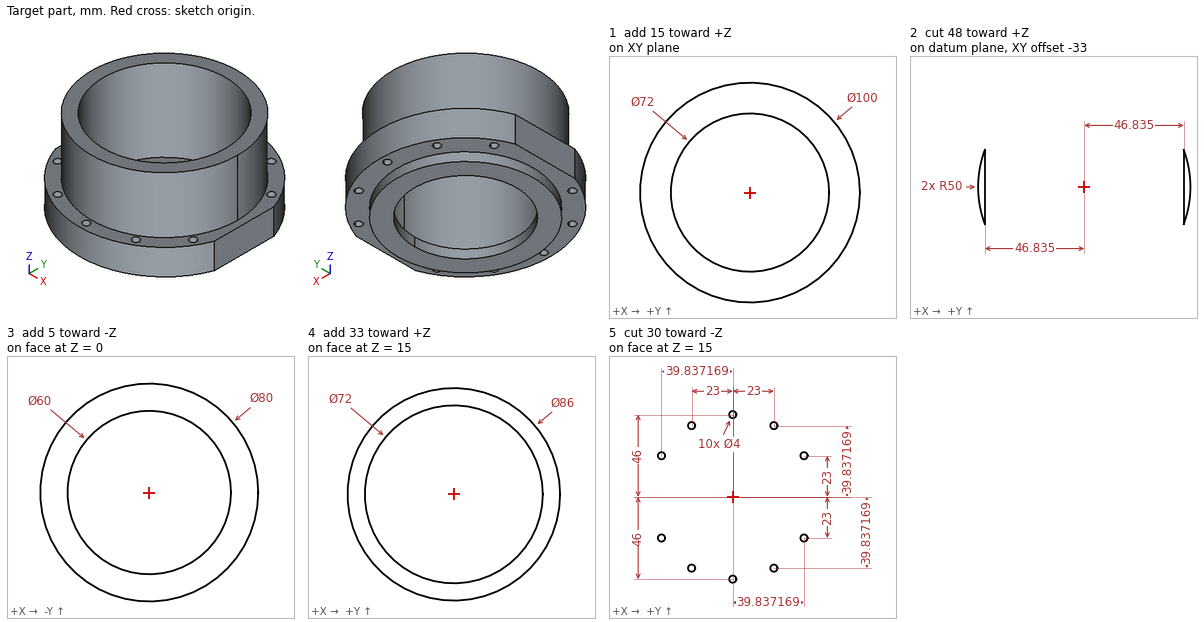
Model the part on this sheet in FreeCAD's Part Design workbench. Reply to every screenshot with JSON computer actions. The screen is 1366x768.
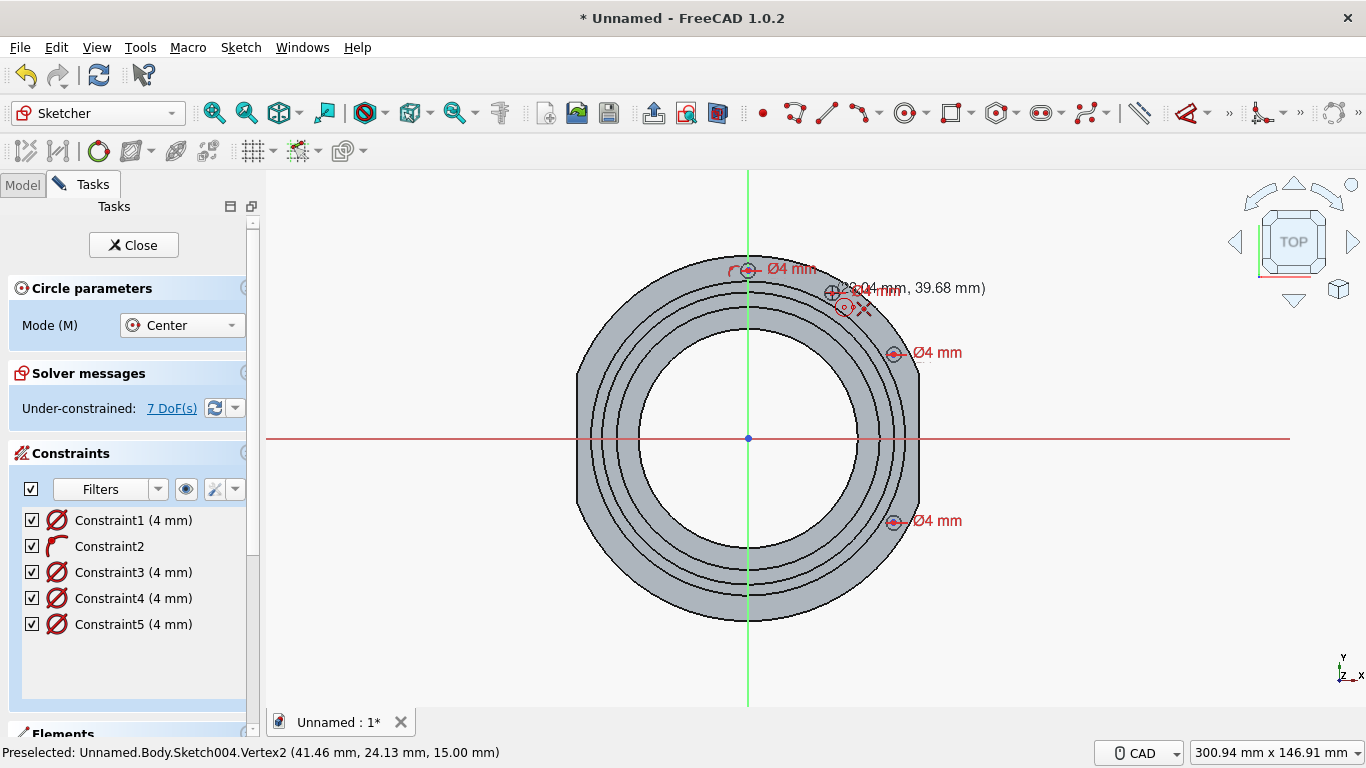
{"action": "scroll", "coordinate": [664, 293], "scroll_direction": "up", "scroll_amount": 6}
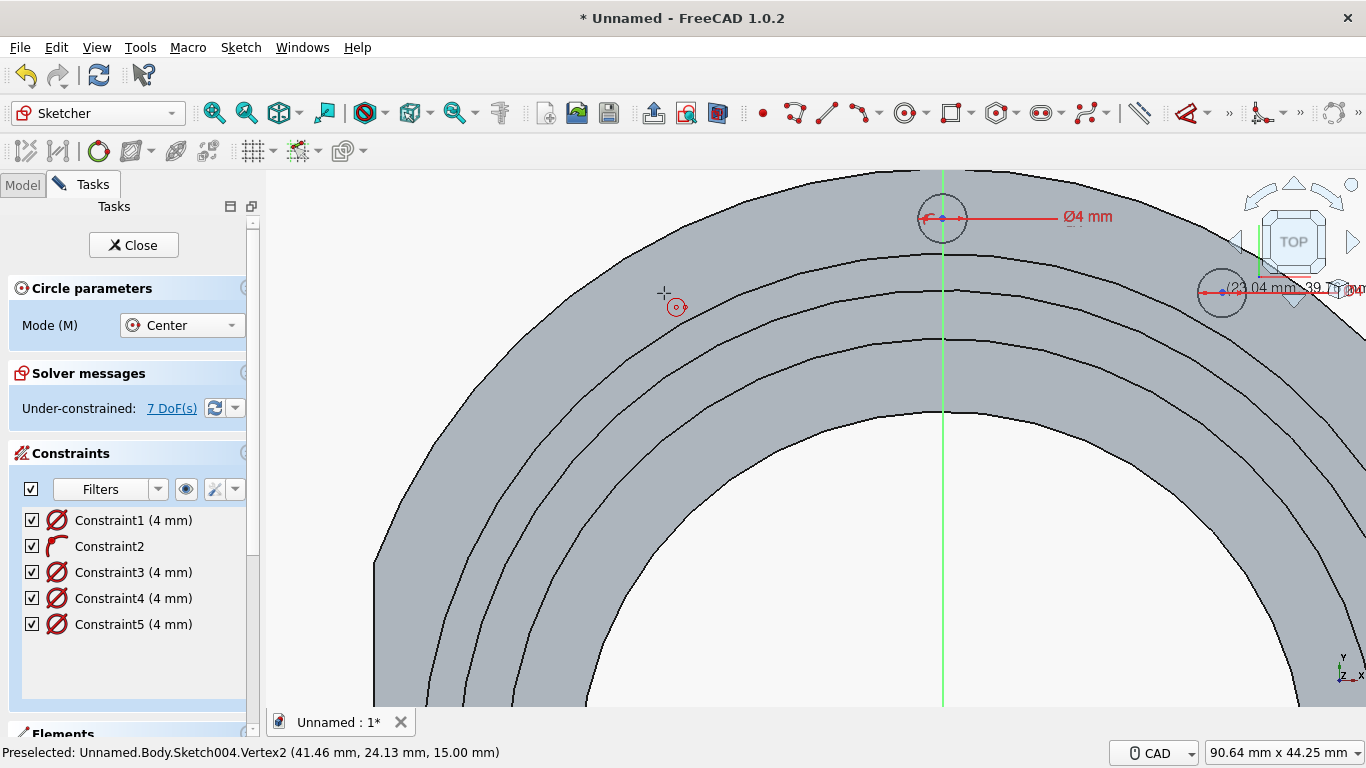
{"action": "left_click", "coordinate": [663, 292]}
{"action": "mouse_move", "coordinate": [681, 275]}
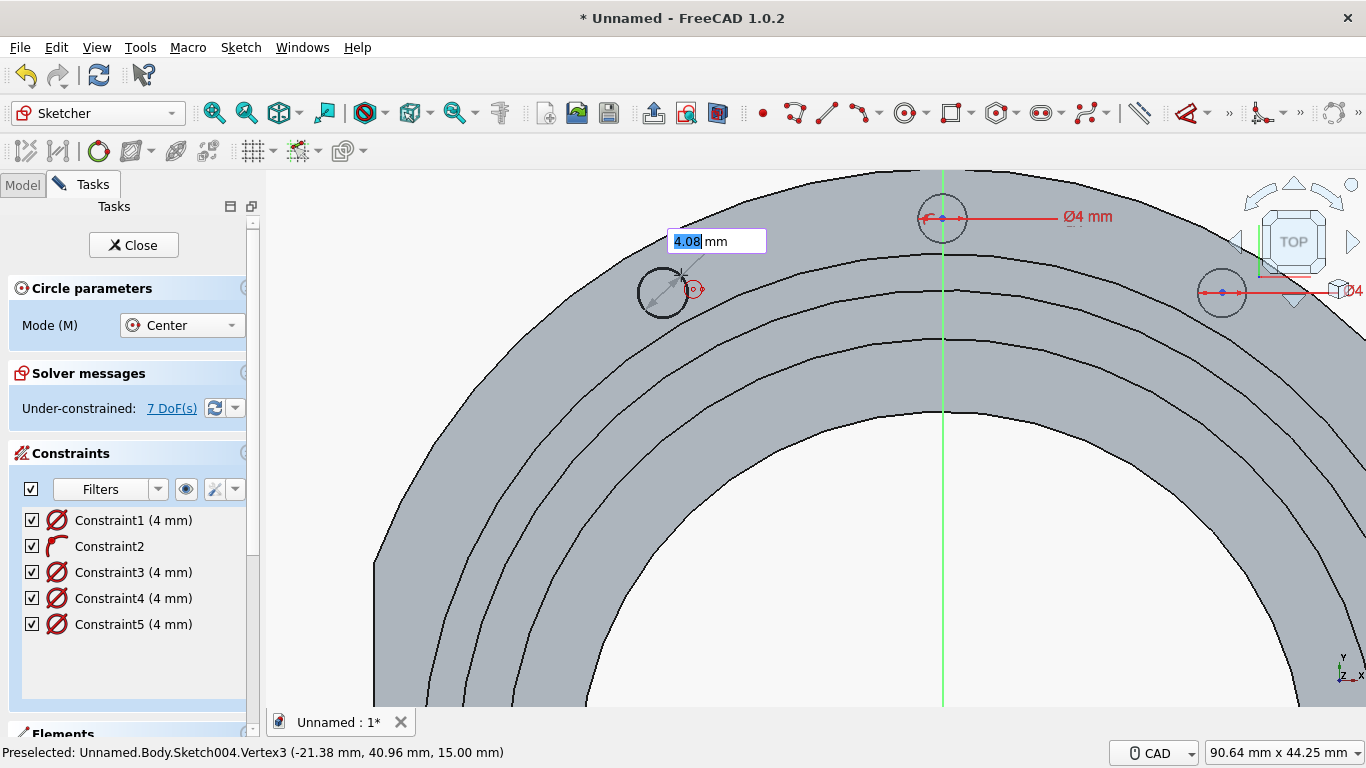
{"action": "type", "text": "4"}
{"action": "key", "text": "Return"}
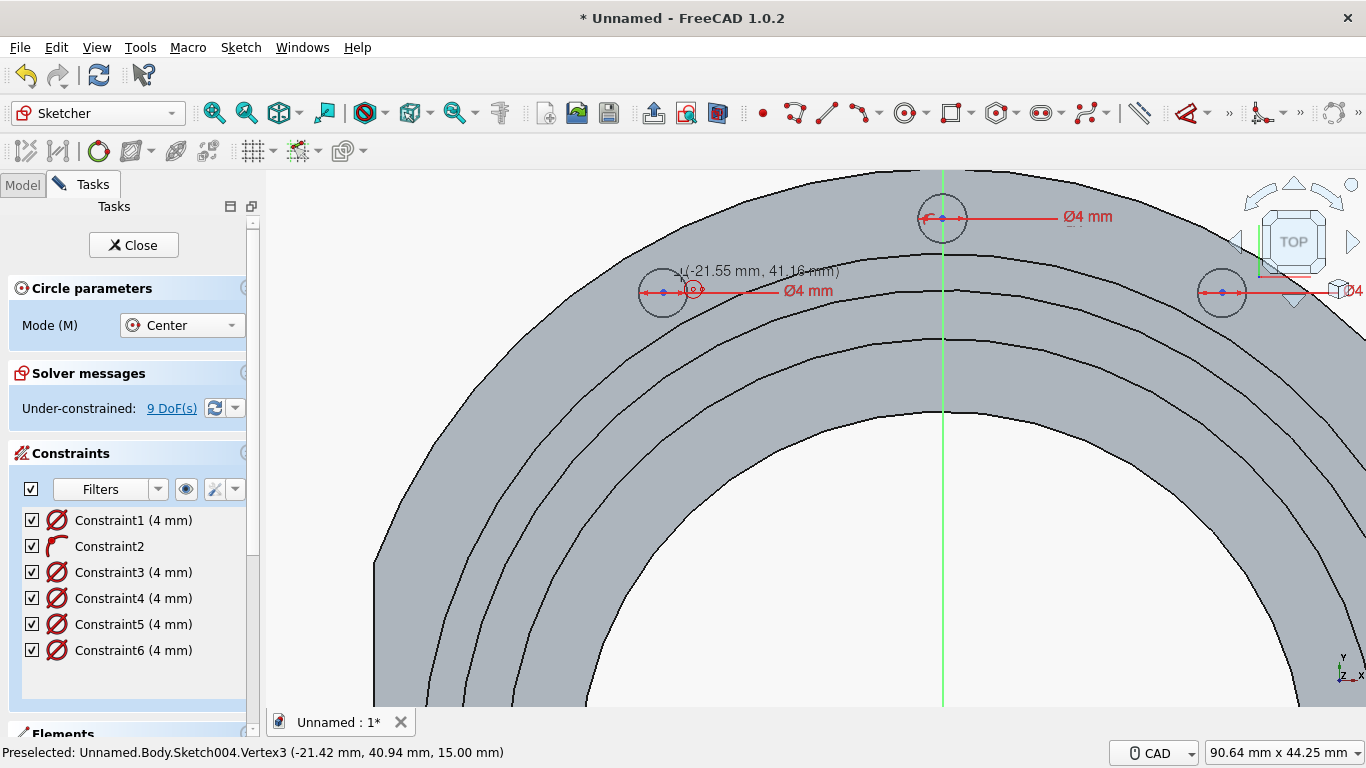
{"action": "left_click", "coordinate": [459, 496]}
{"action": "mouse_move", "coordinate": [476, 479]}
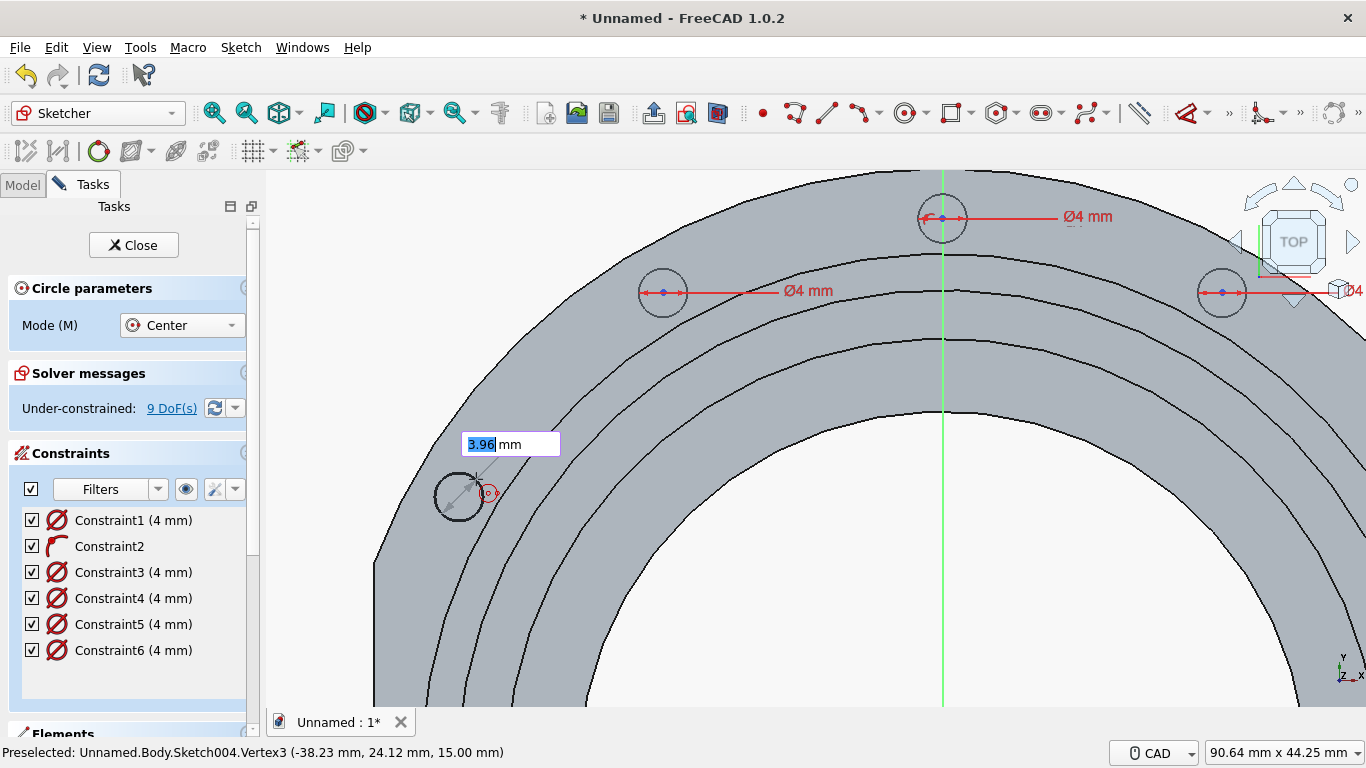
{"action": "type", "text": "4"}
{"action": "key", "text": "Return"}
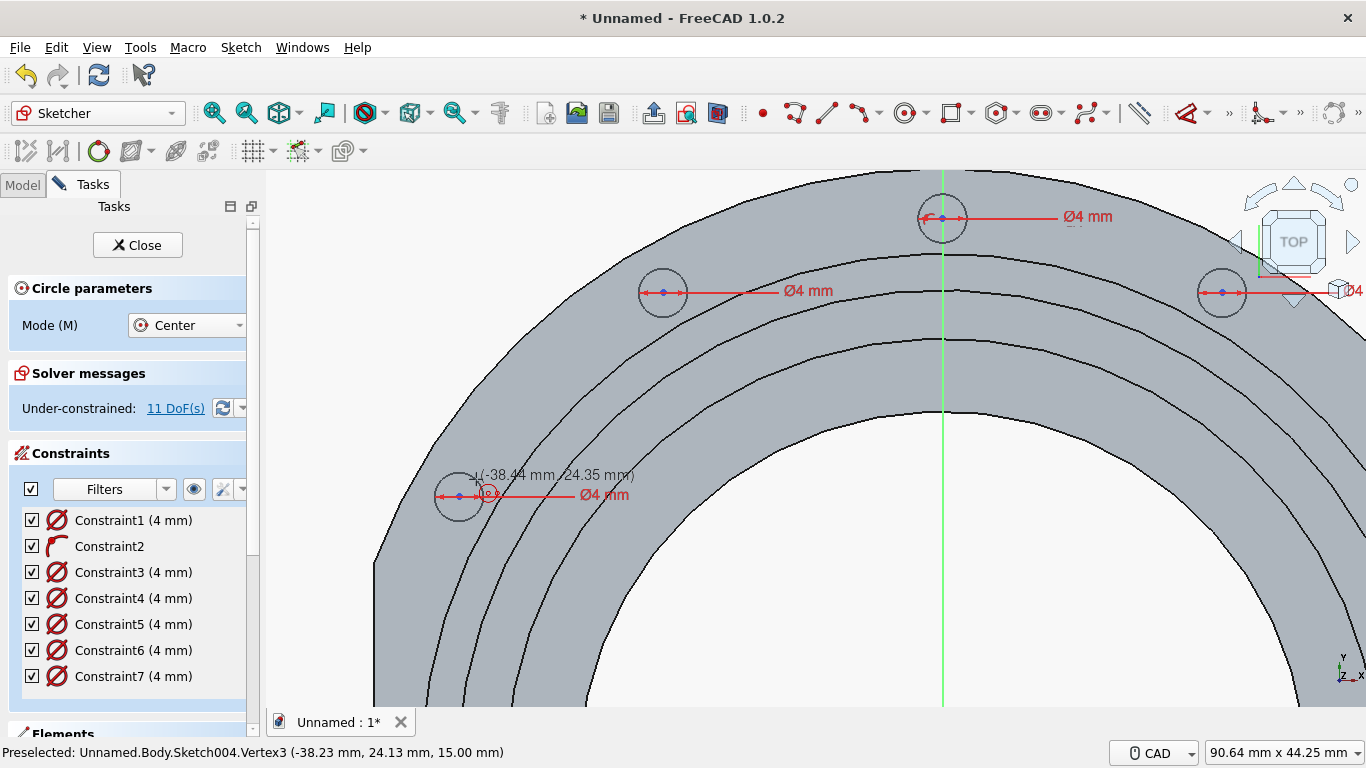
{"action": "scroll", "coordinate": [663, 293], "scroll_direction": "down", "scroll_amount": 6}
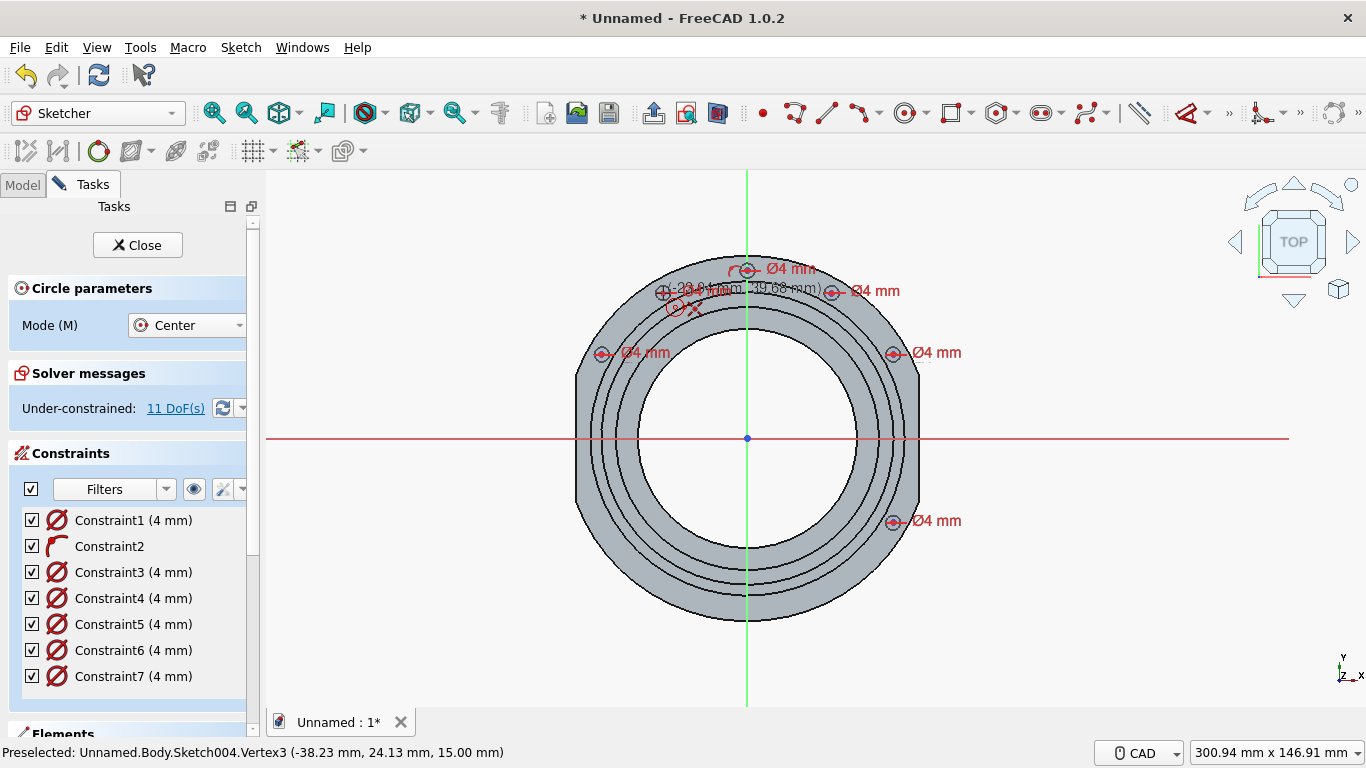
{"action": "scroll", "coordinate": [832, 584], "scroll_direction": "up", "scroll_amount": 6}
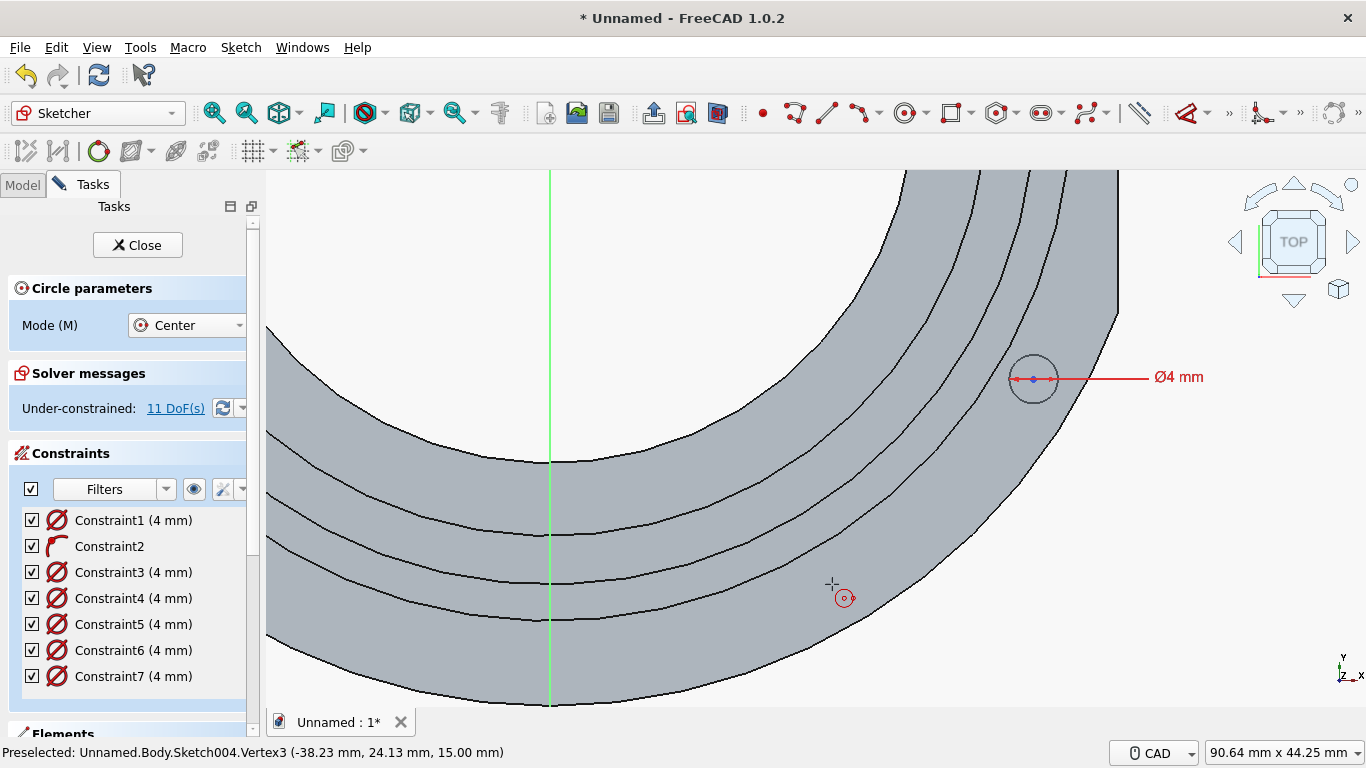
{"action": "left_click", "coordinate": [829, 583]}
{"action": "mouse_move", "coordinate": [846, 565]}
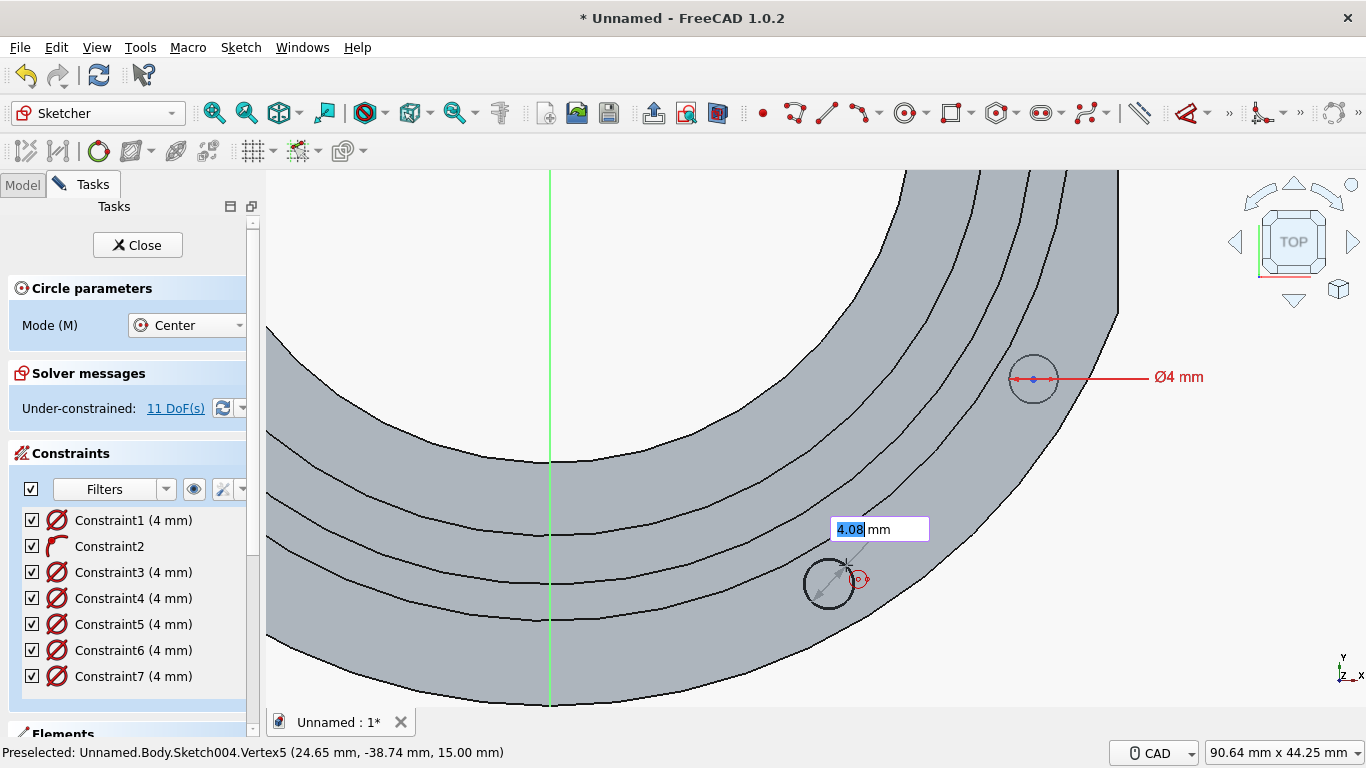
{"action": "type", "text": "4"}
{"action": "key", "text": "Return"}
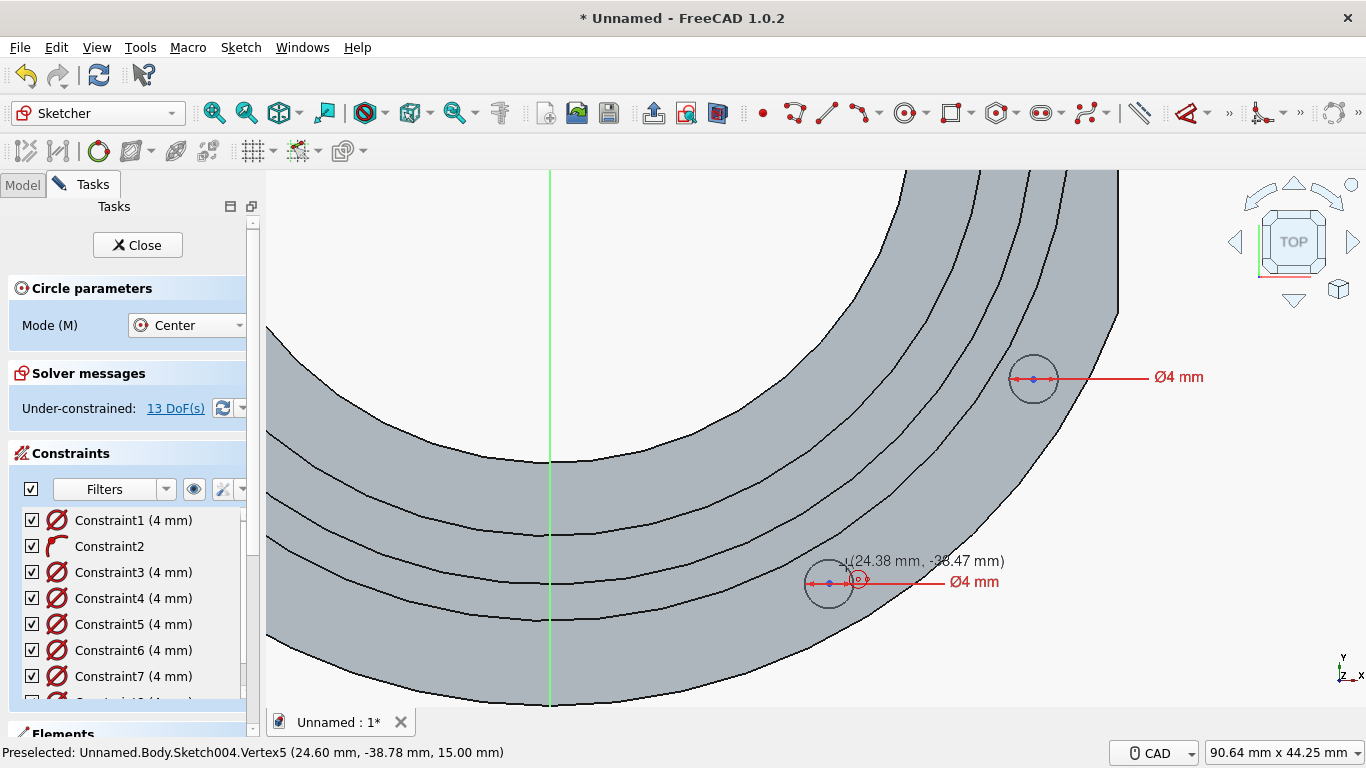
{"action": "left_click", "coordinate": [550, 657]}
{"action": "mouse_move", "coordinate": [567, 640]}